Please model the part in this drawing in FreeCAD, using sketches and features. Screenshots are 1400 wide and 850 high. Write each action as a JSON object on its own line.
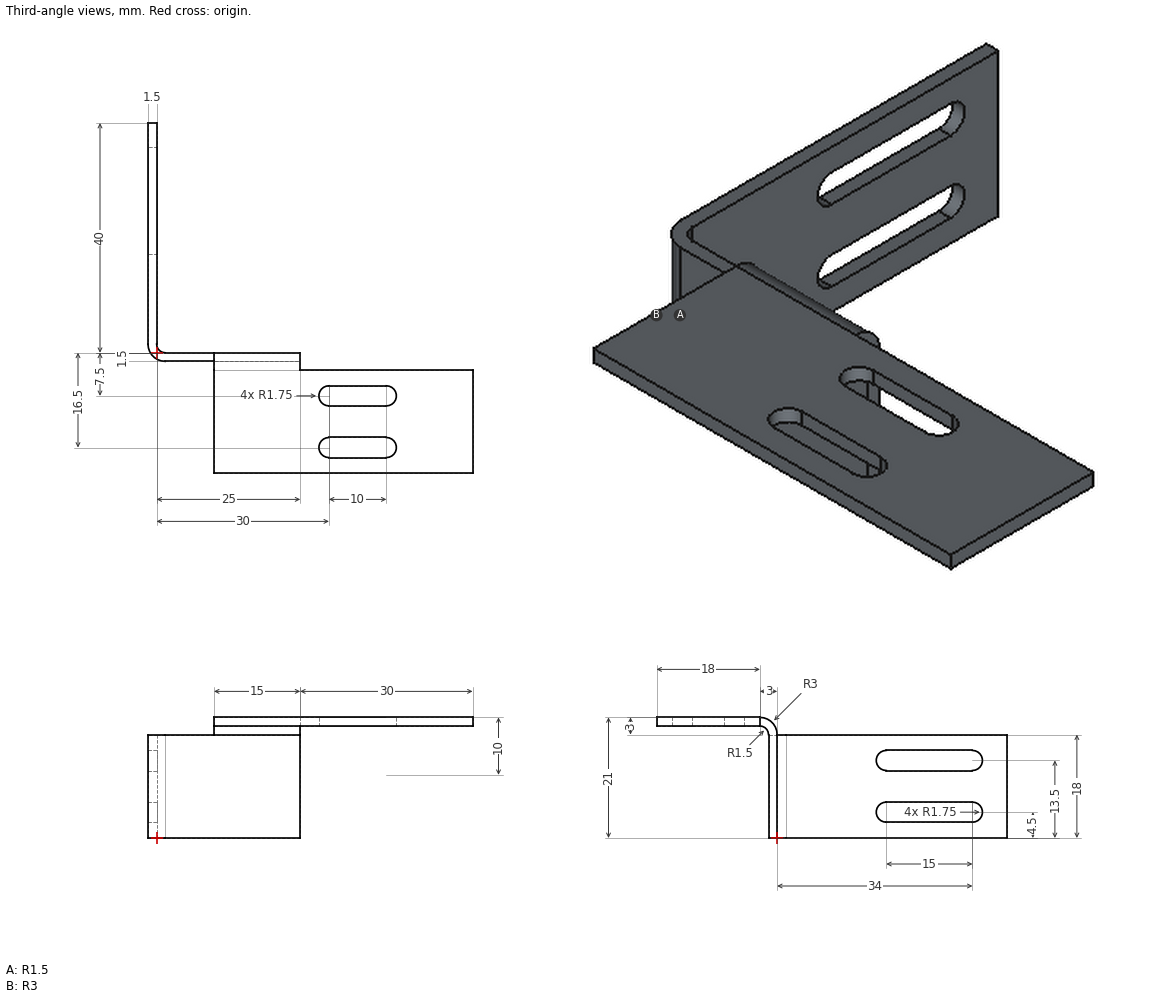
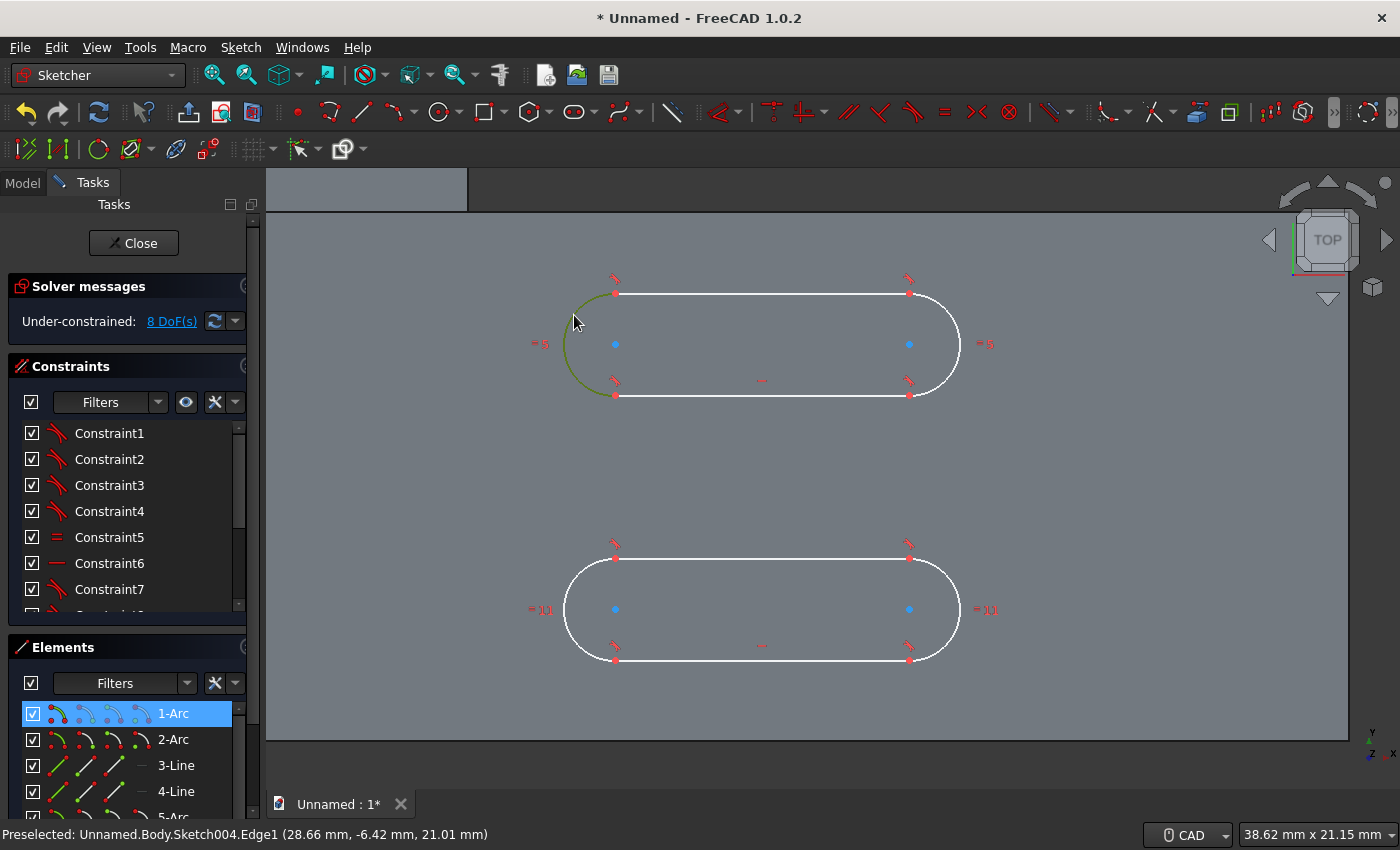
{"action": "left_click", "coordinate": [574, 580]}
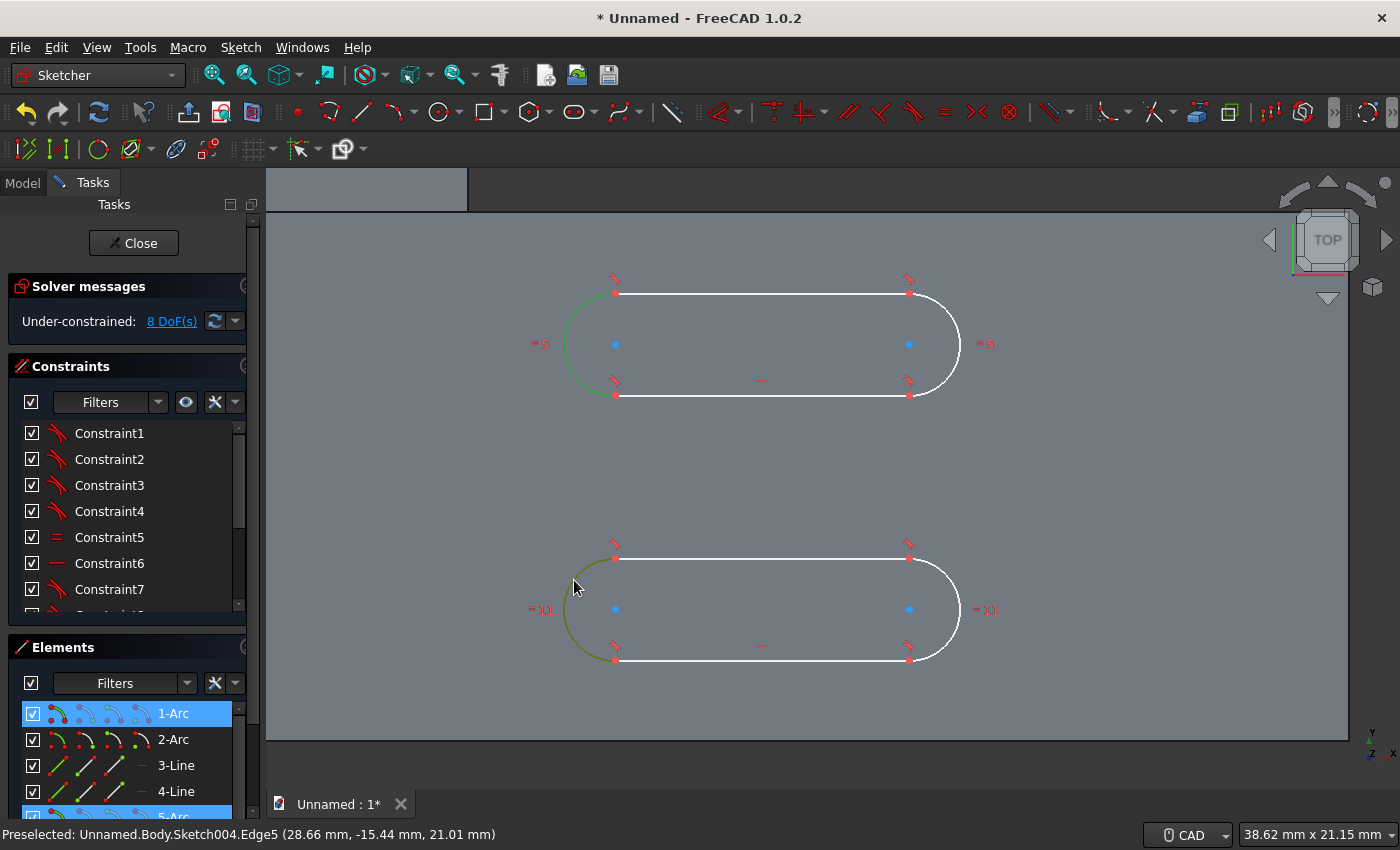
{"action": "key", "text": "e"}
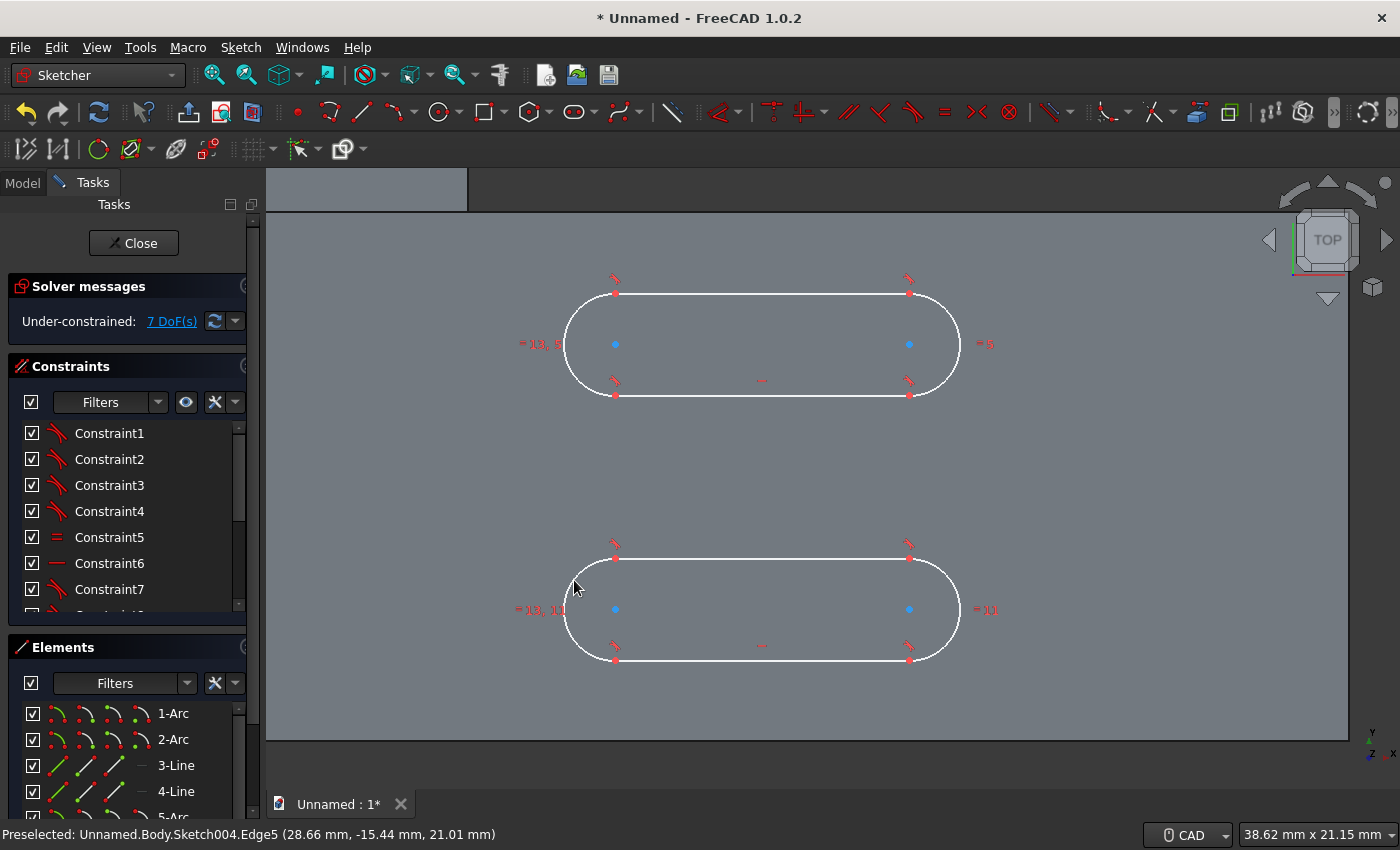
{"action": "key", "text": "d"}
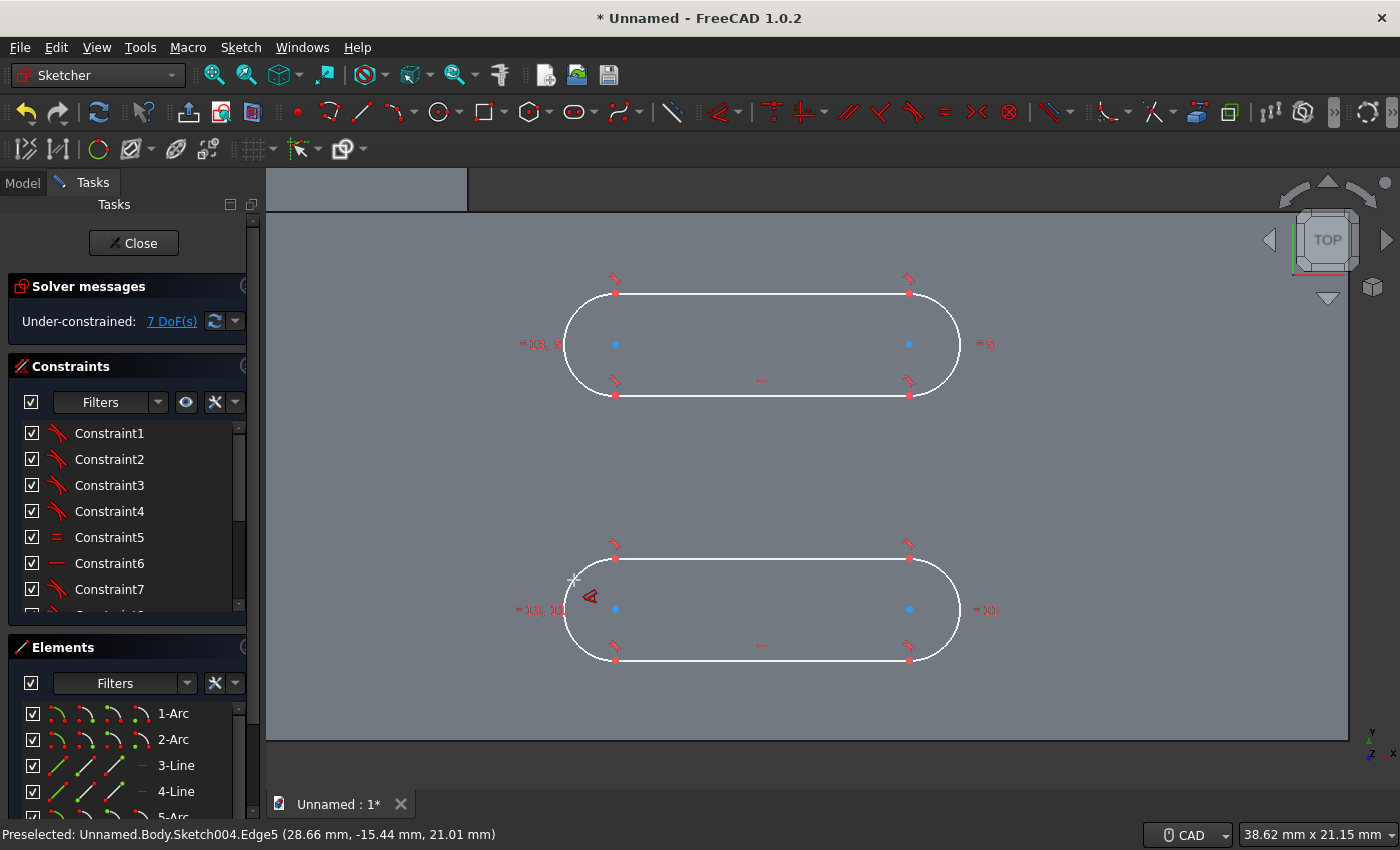
{"action": "left_click", "coordinate": [574, 315]}
{"action": "left_click", "coordinate": [548, 296]}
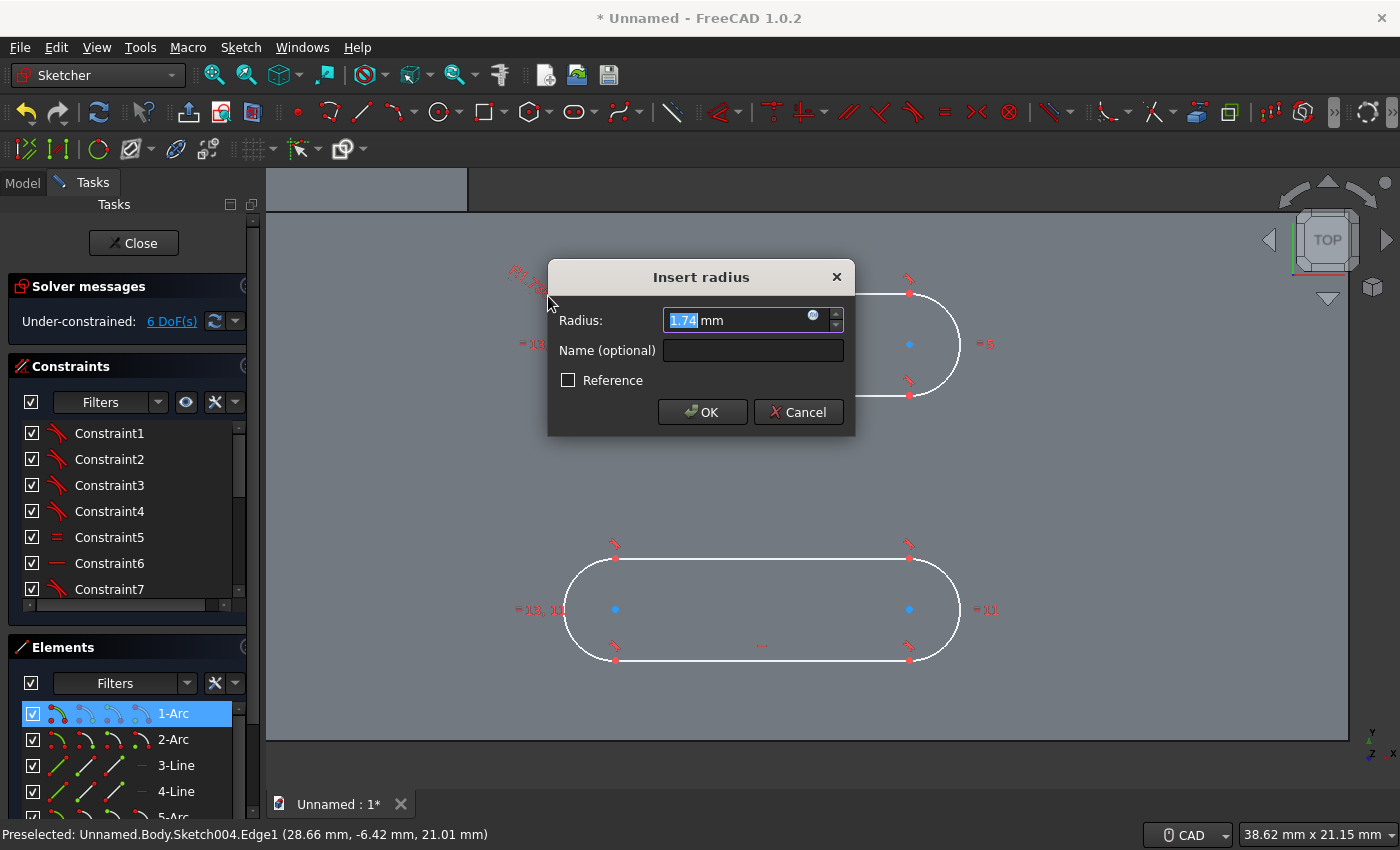
{"action": "type", "text": "1.75"}
{"action": "key", "text": "Return"}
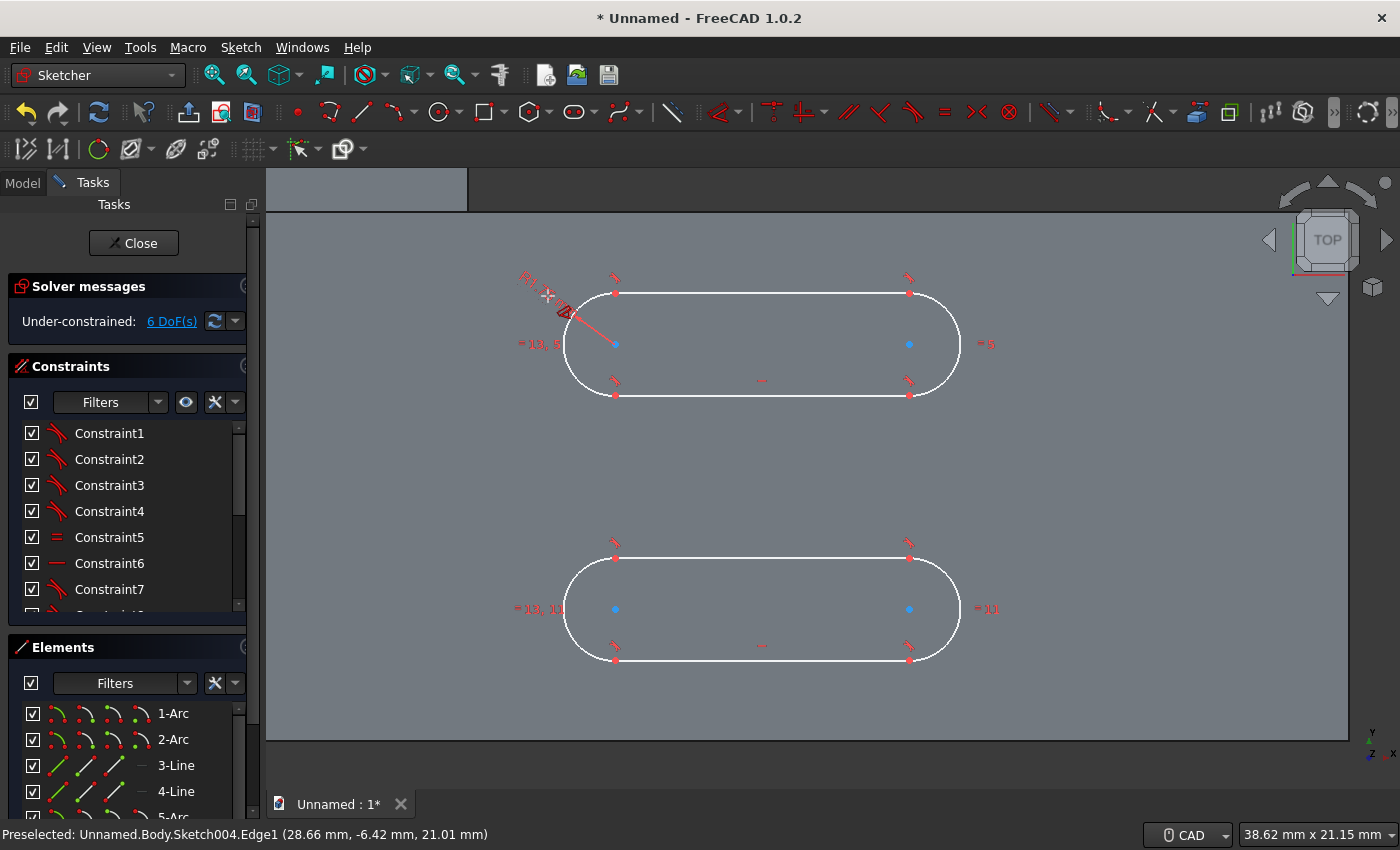
{"action": "left_click", "coordinate": [703, 293]}
{"action": "left_click", "coordinate": [762, 259]}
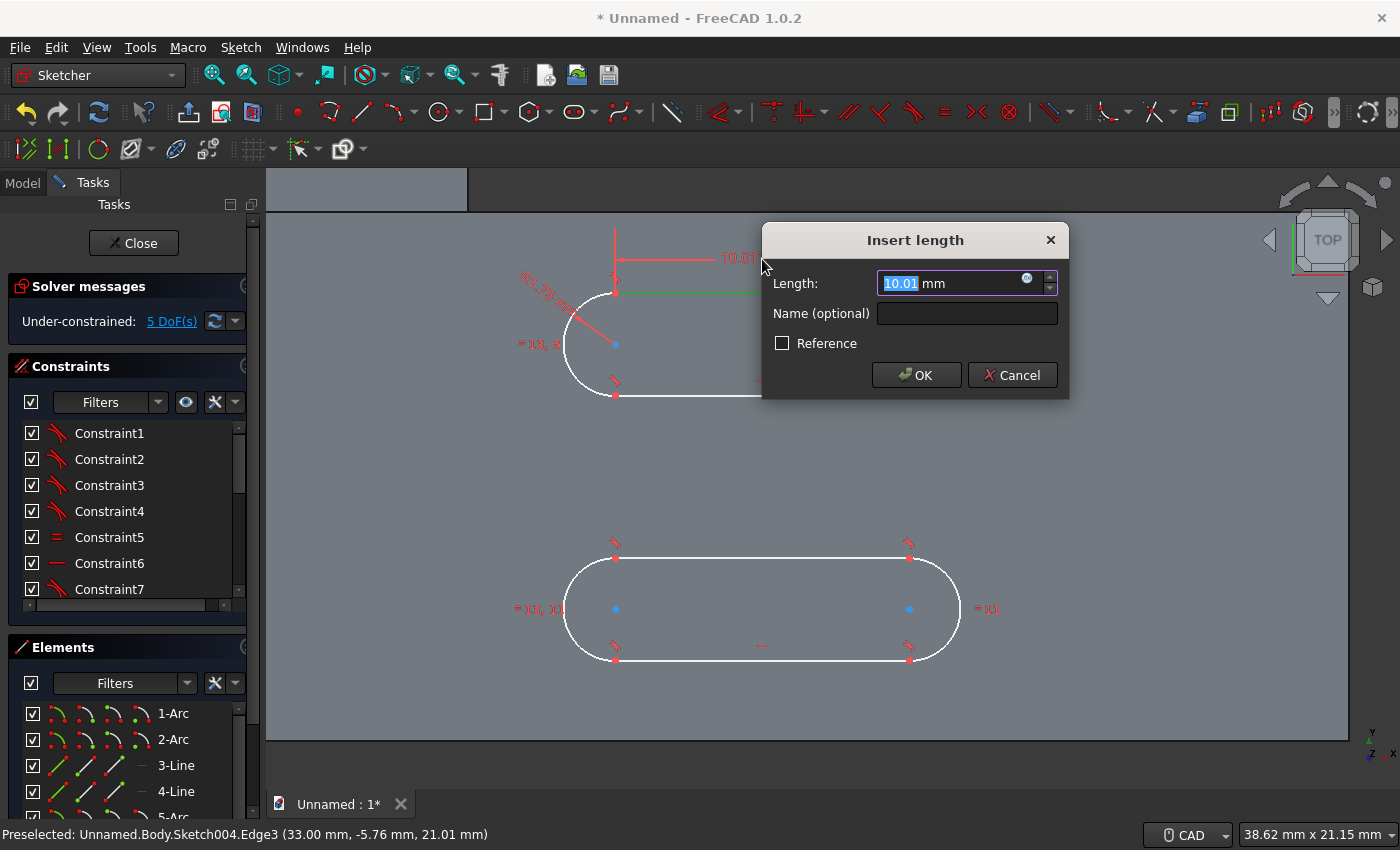
{"action": "type", "text": "10"}
{"action": "key", "text": "Return"}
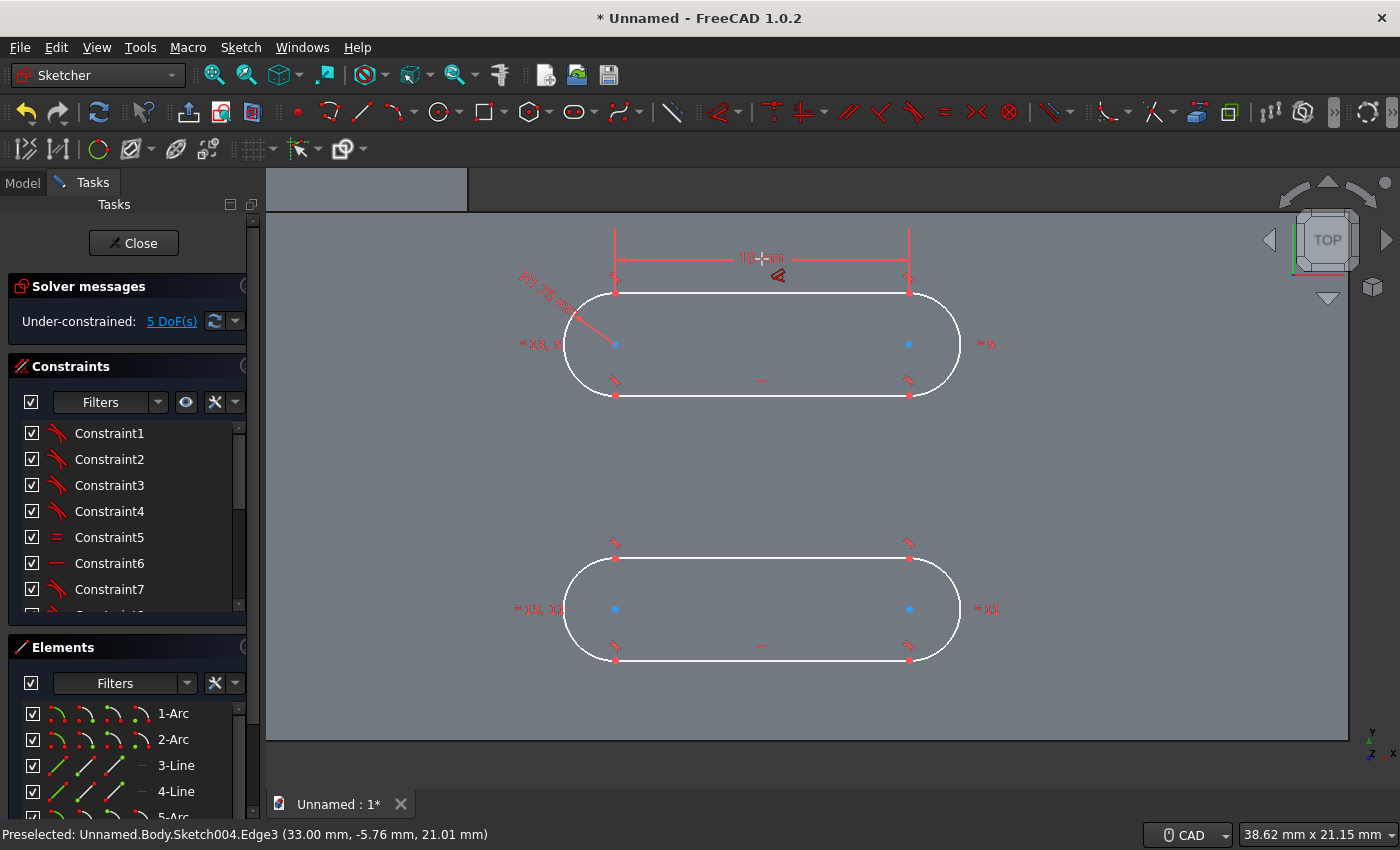
{"action": "left_click", "coordinate": [703, 558]}
{"action": "left_click", "coordinate": [762, 592]}